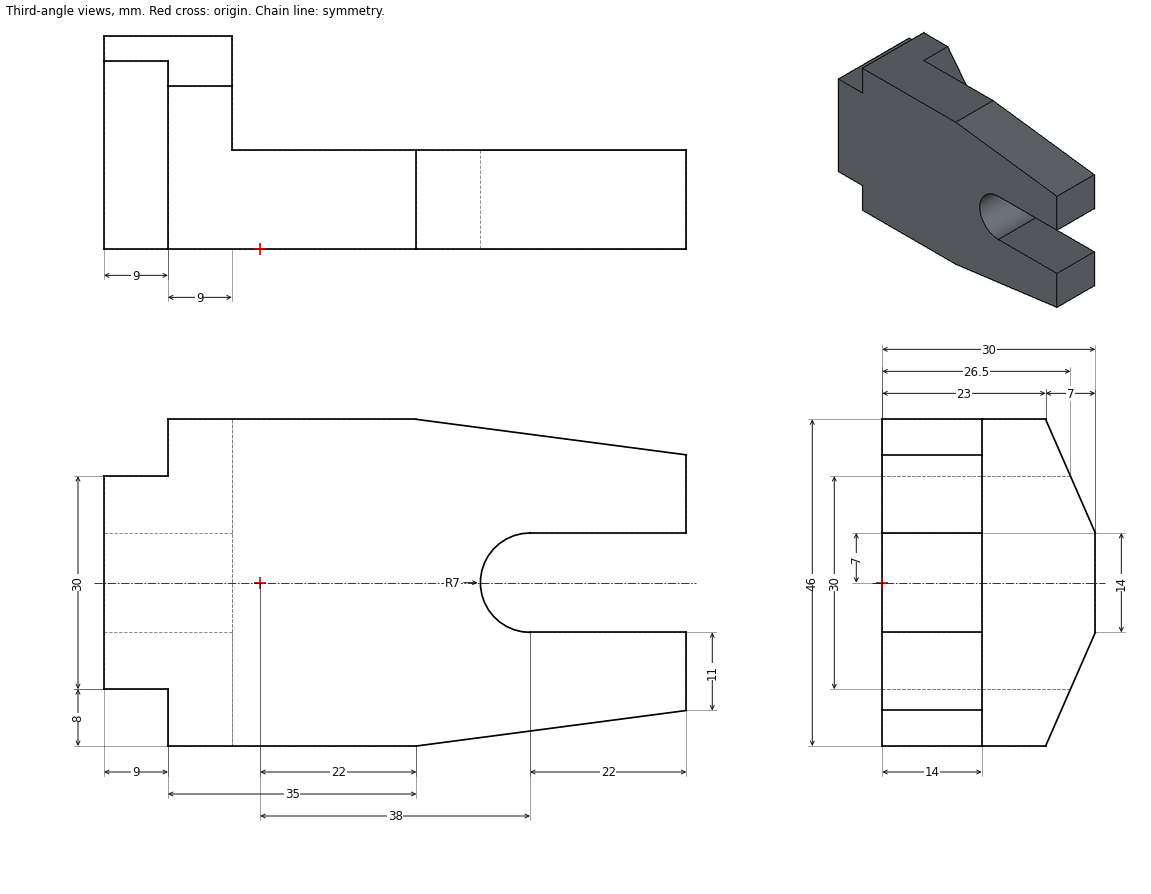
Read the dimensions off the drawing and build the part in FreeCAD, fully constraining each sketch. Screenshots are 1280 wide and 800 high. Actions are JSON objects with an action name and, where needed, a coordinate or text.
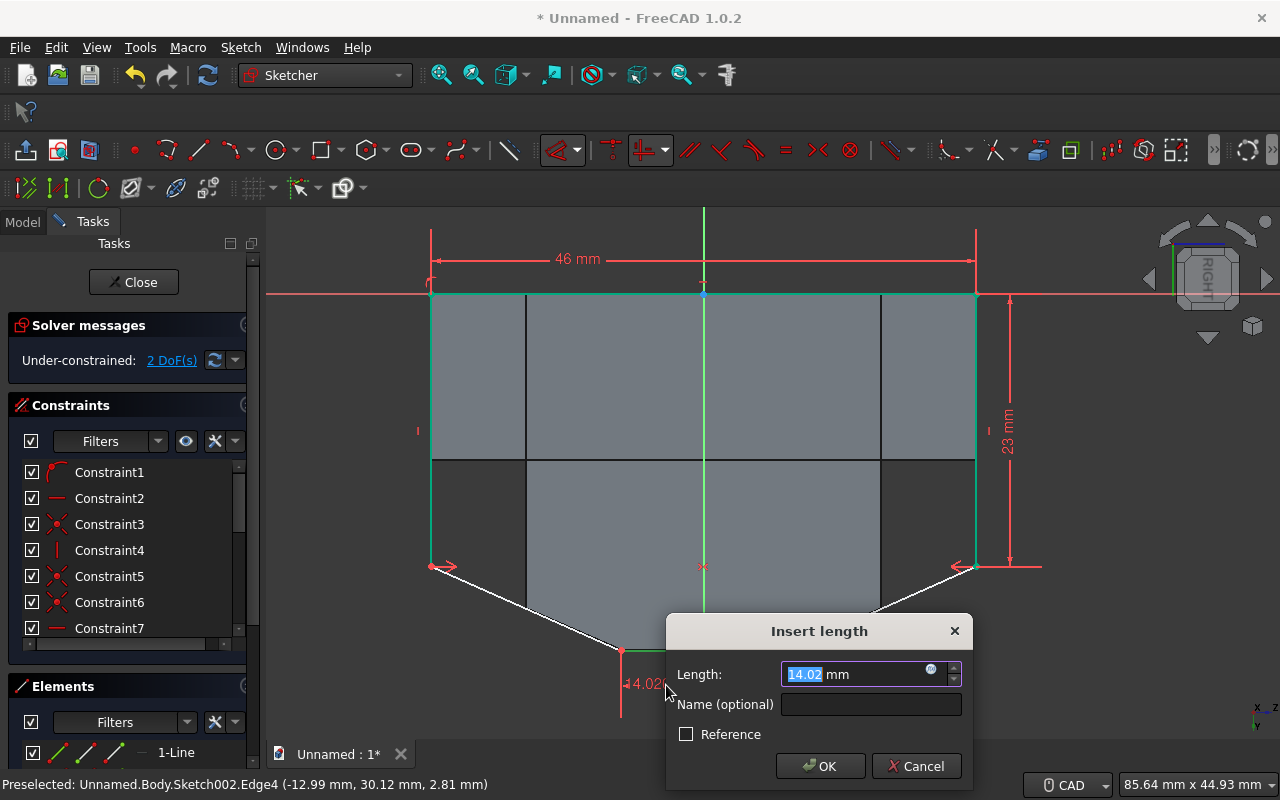
{"action": "type", "text": "14"}
{"action": "key", "text": "Return"}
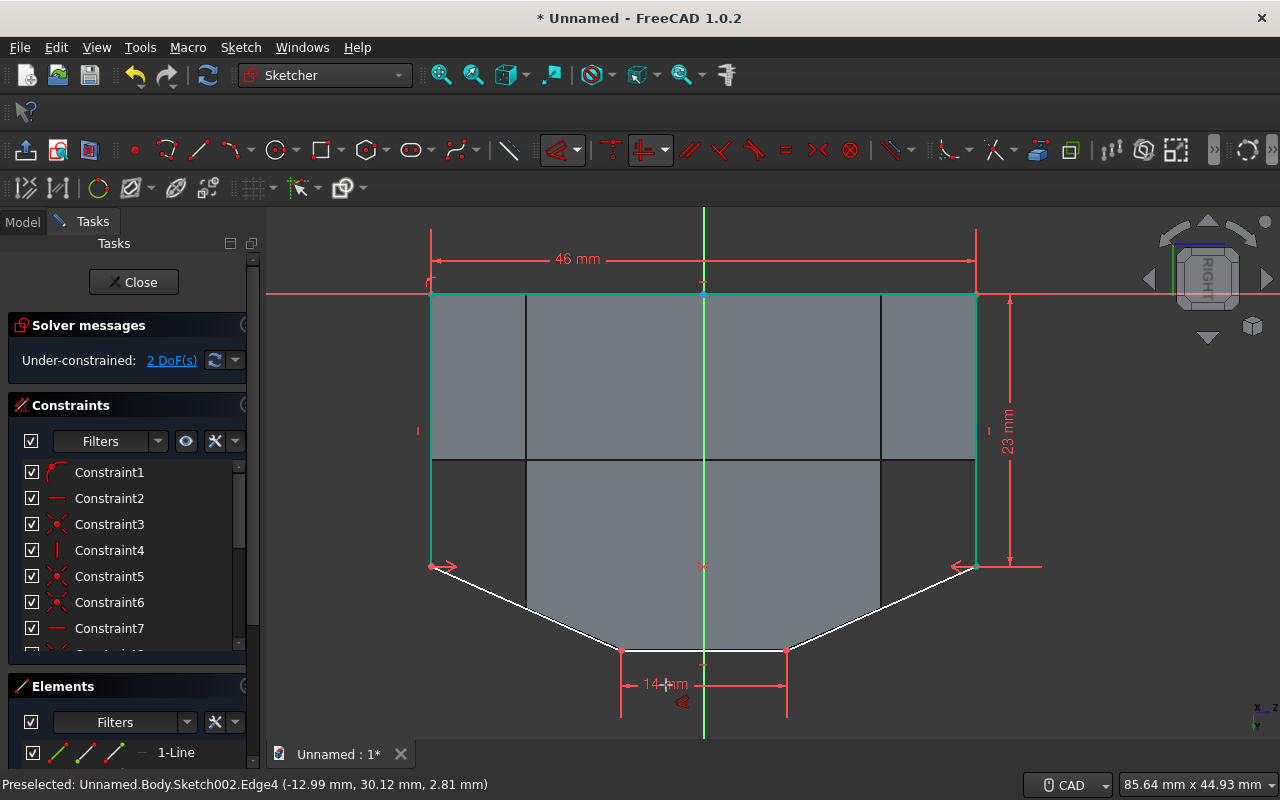
{"action": "left_click", "coordinate": [787, 651]}
{"action": "left_click", "coordinate": [745, 685]}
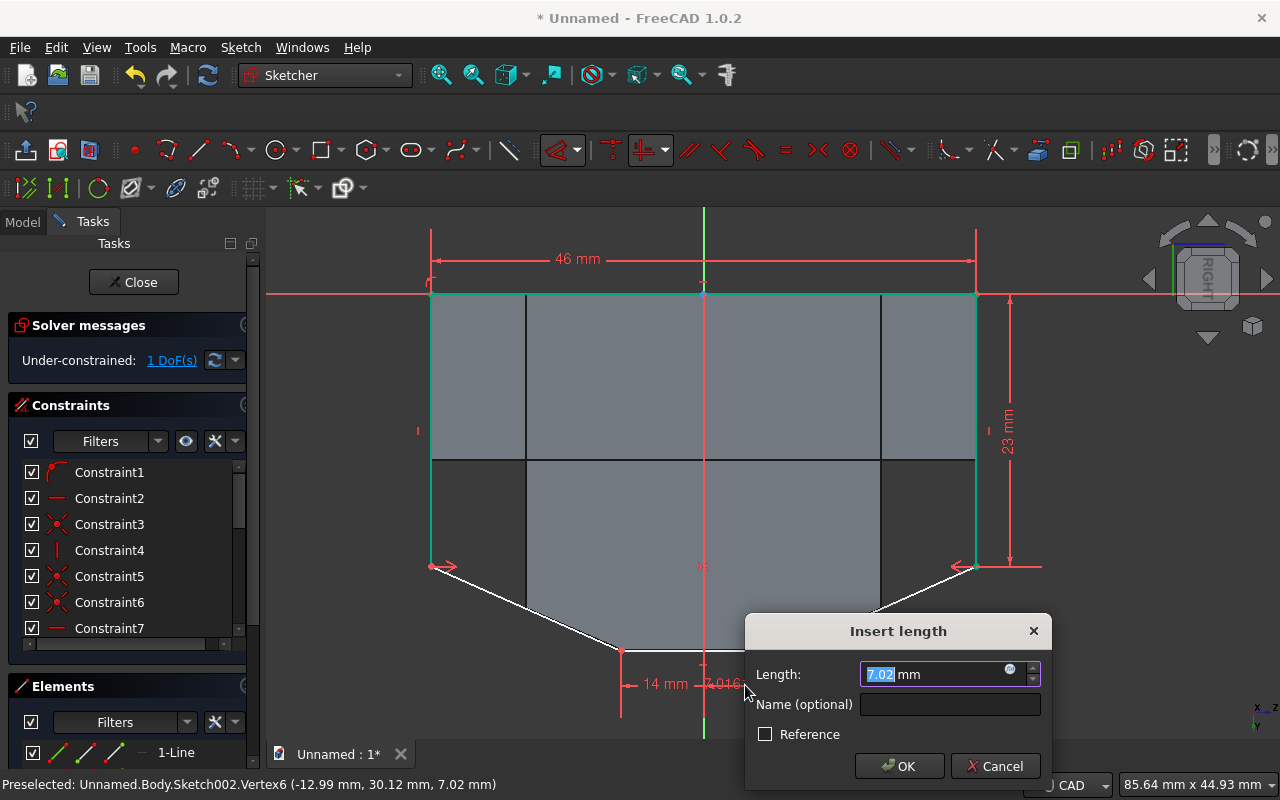
{"action": "type", "text": "7"}
{"action": "key", "text": "Return"}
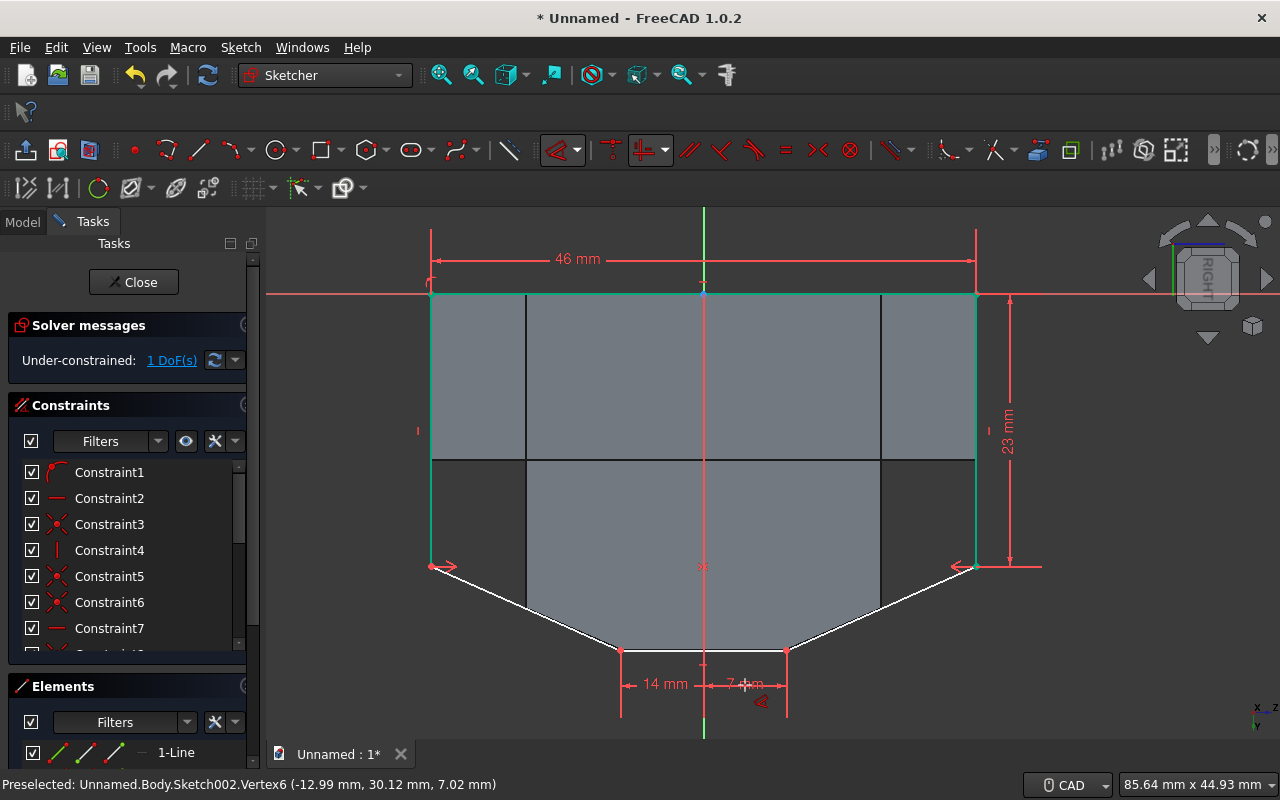
{"action": "left_click", "coordinate": [919, 592]}
{"action": "left_click", "coordinate": [1010, 609]}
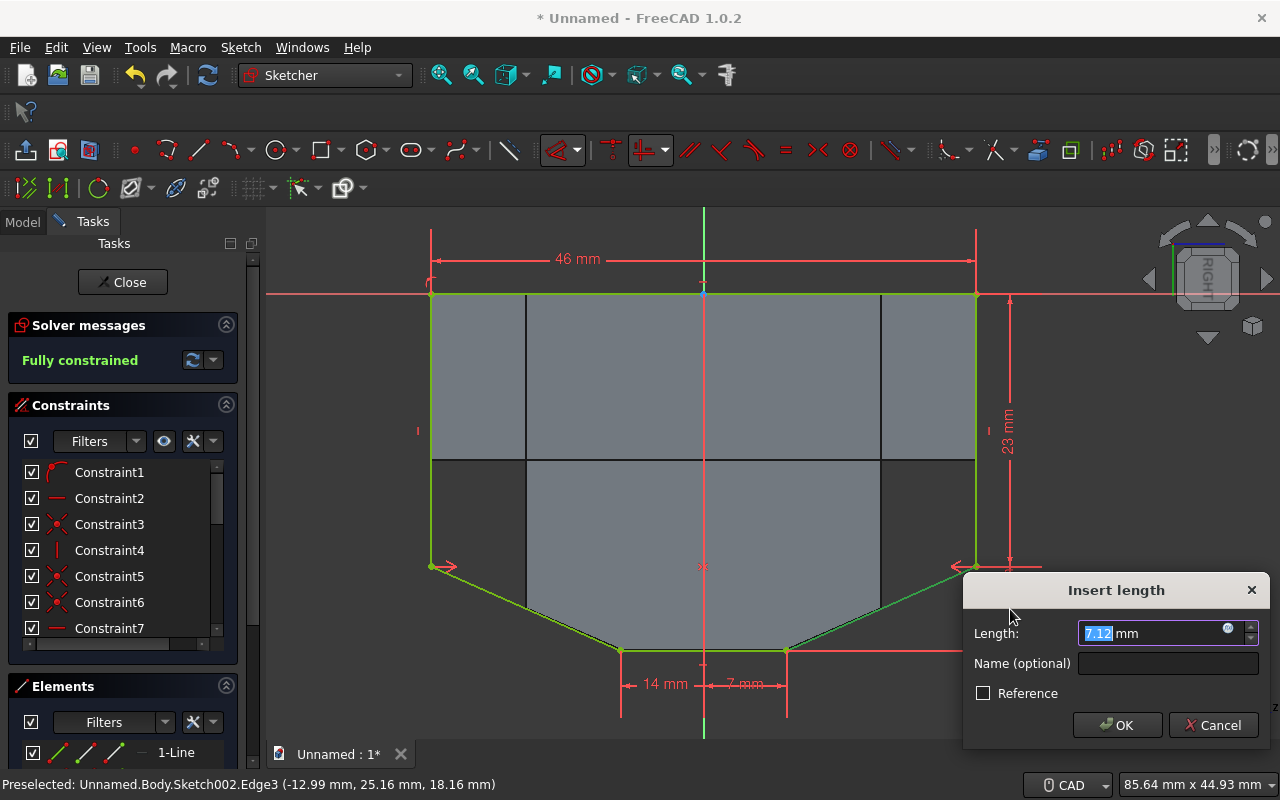
{"action": "type", "text": "7"}
{"action": "key", "text": "Return"}
{"action": "key", "text": "Escape"}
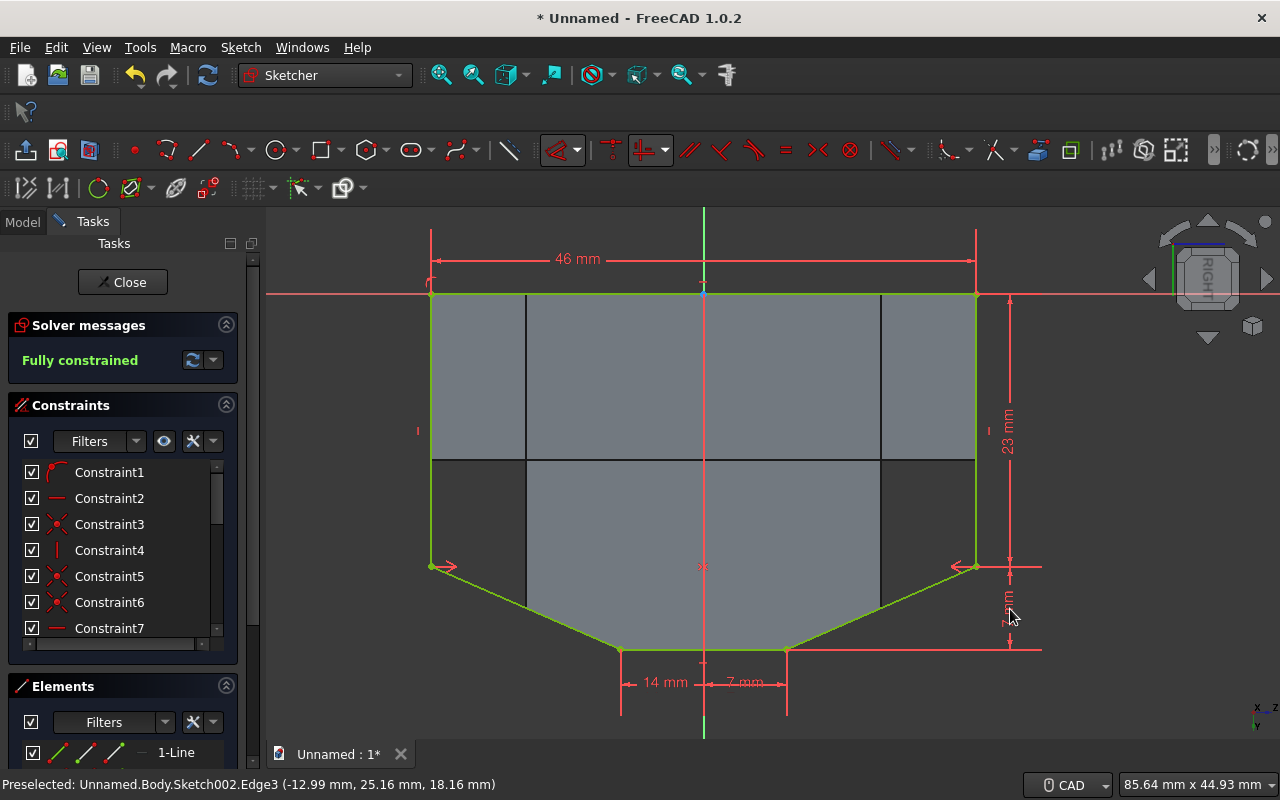
{"action": "left_click", "coordinate": [123, 282]}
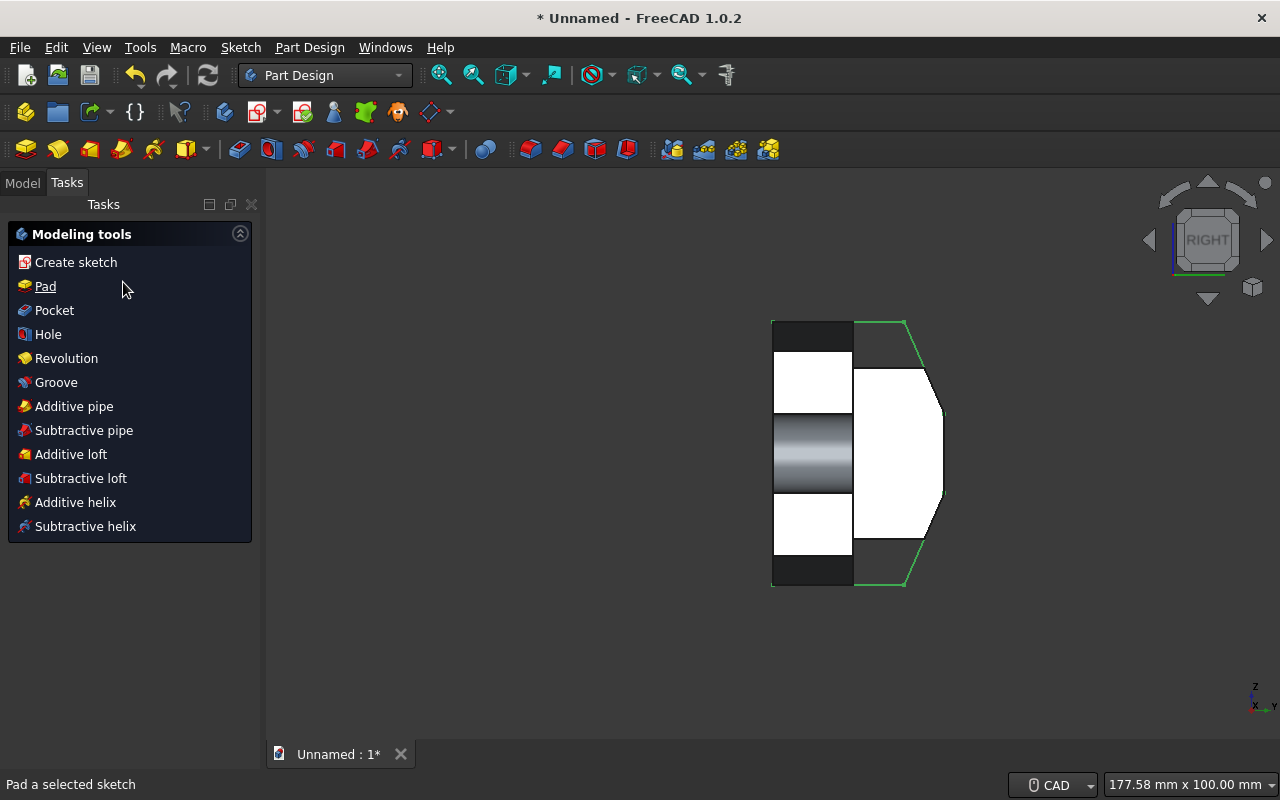
{"action": "left_click", "coordinate": [26, 150]}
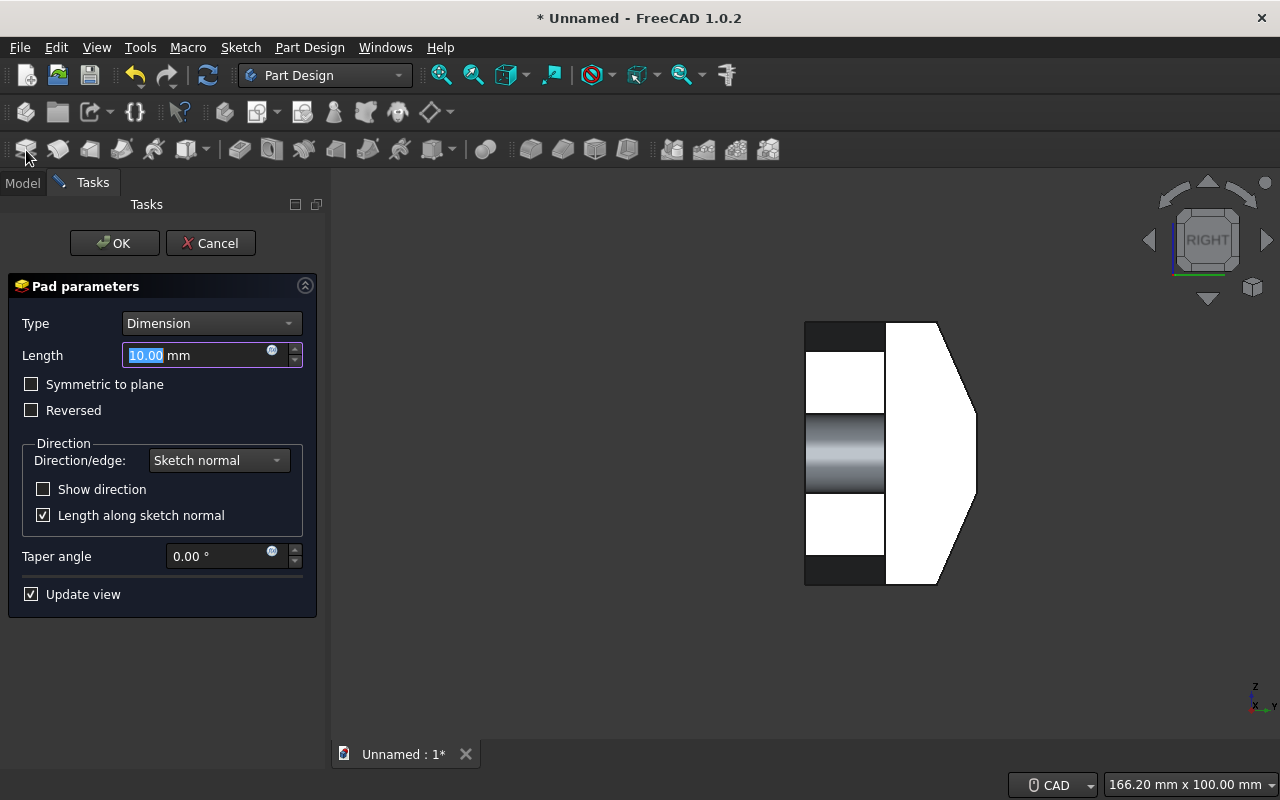
{"action": "type", "text": "9"}
{"action": "key", "text": "Tab"}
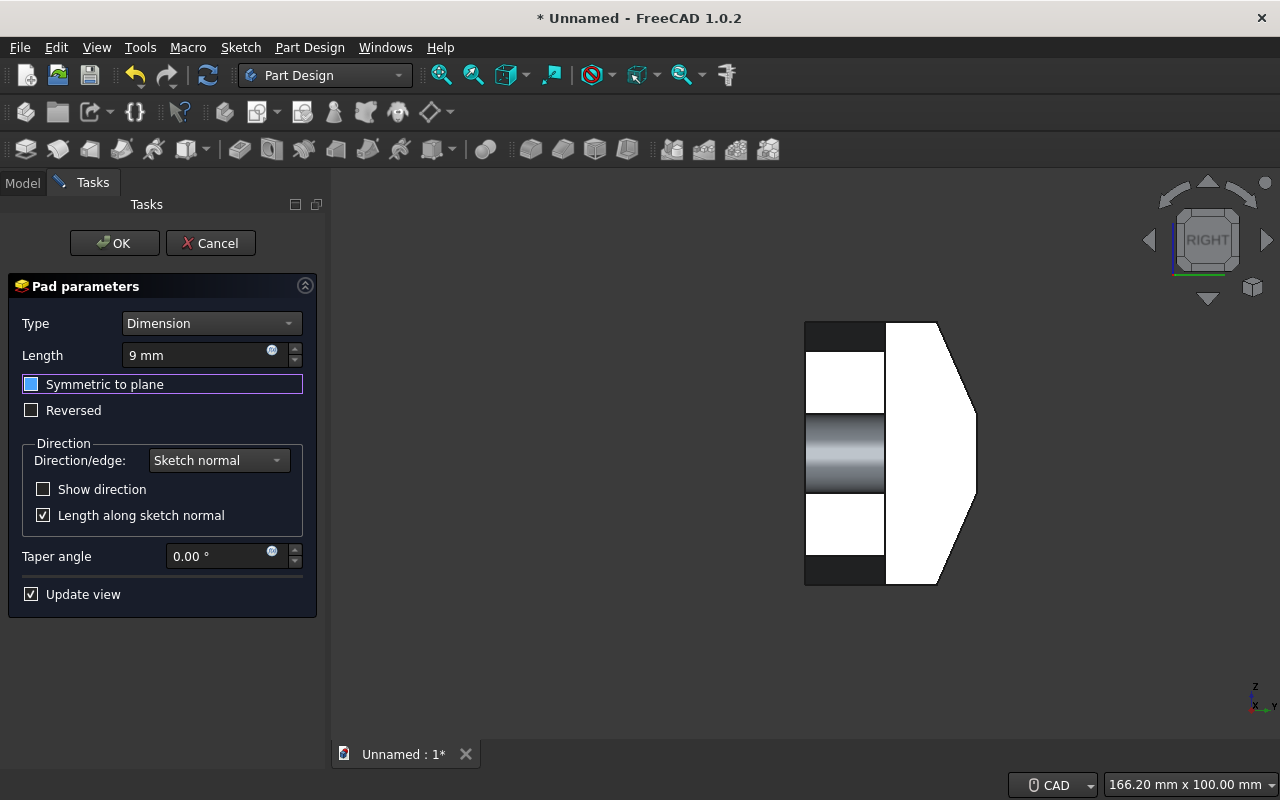
{"action": "left_click", "coordinate": [115, 243]}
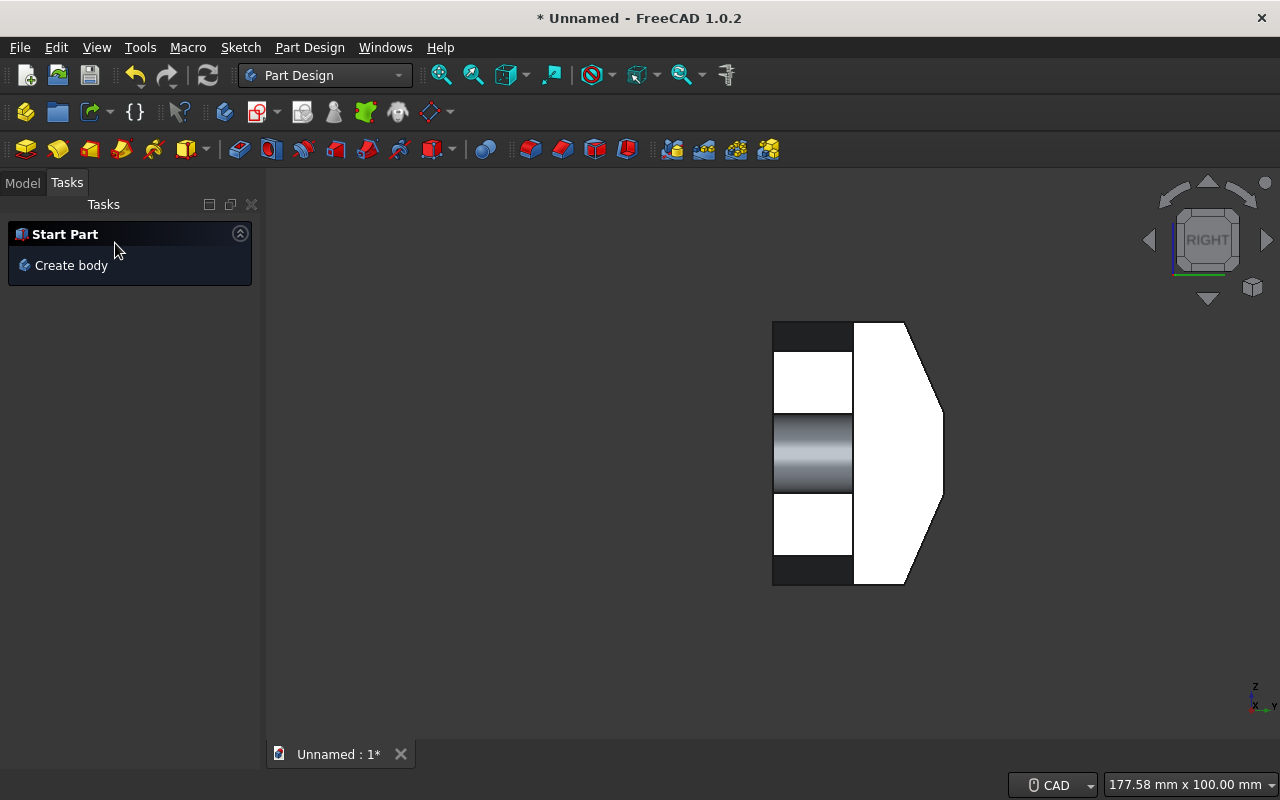
{"action": "key", "text": "0"}